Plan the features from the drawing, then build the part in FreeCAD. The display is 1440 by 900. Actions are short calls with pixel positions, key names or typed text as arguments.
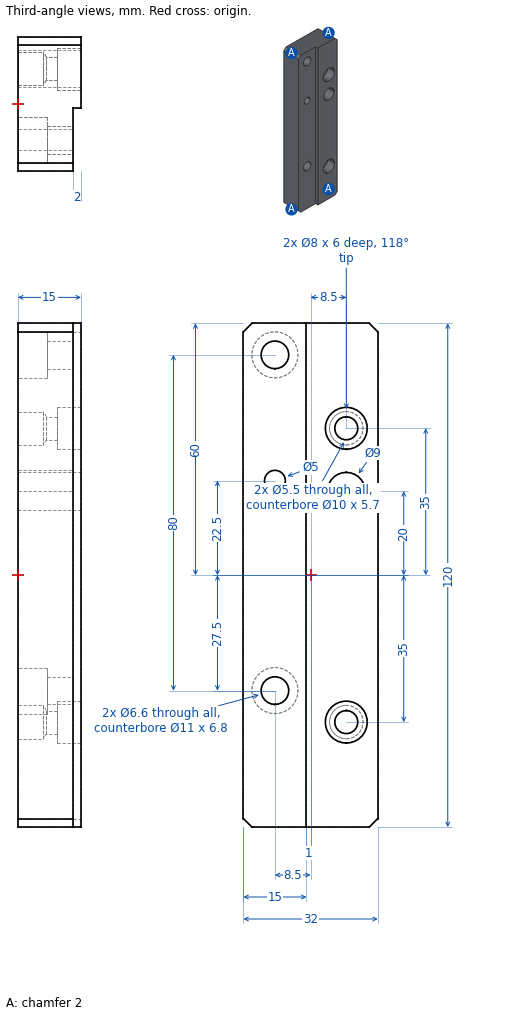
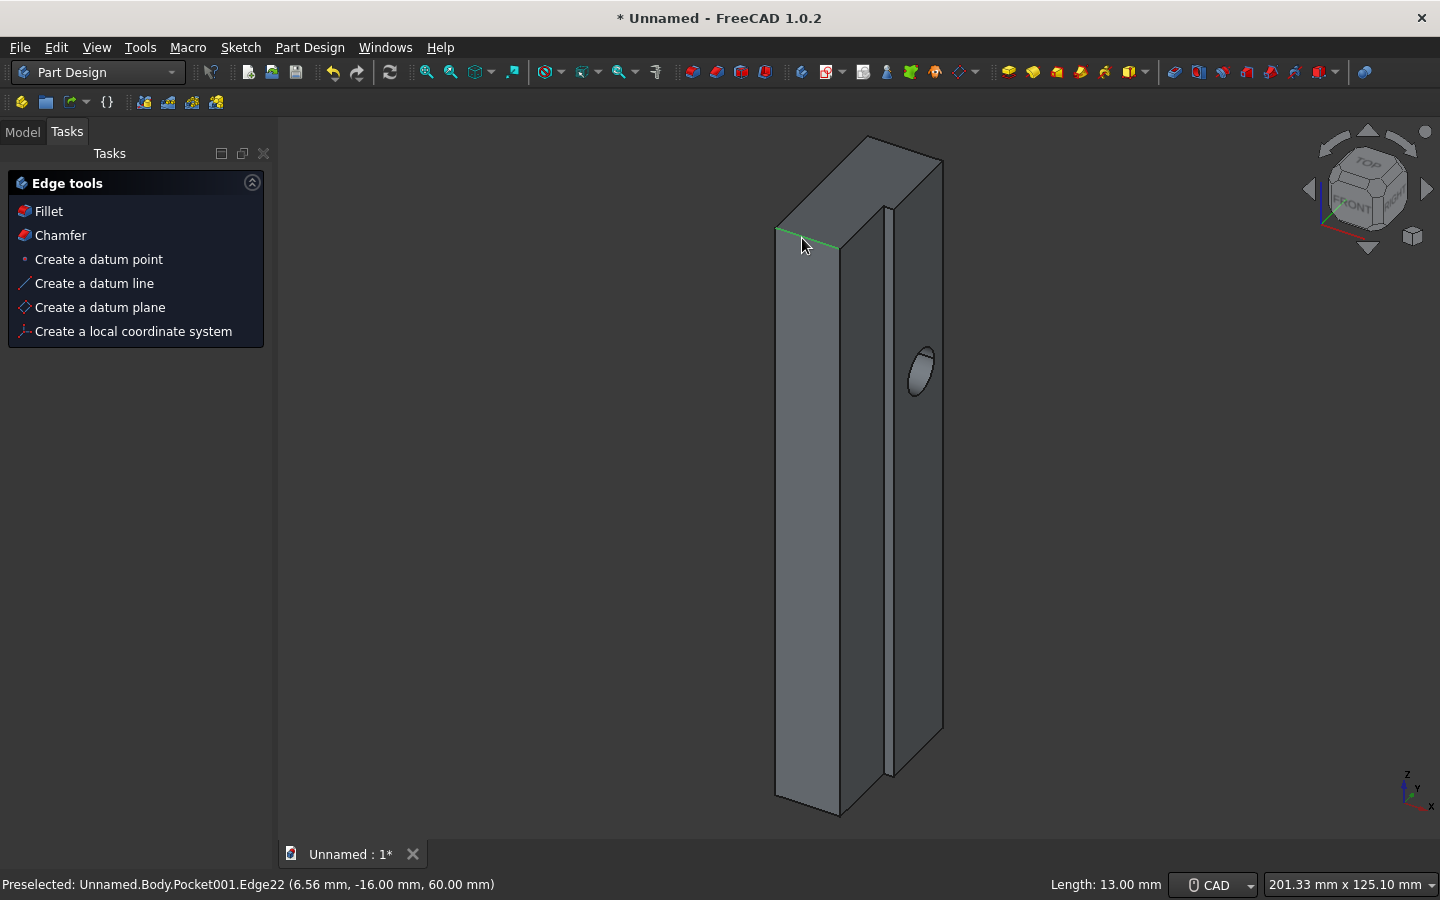
key(0)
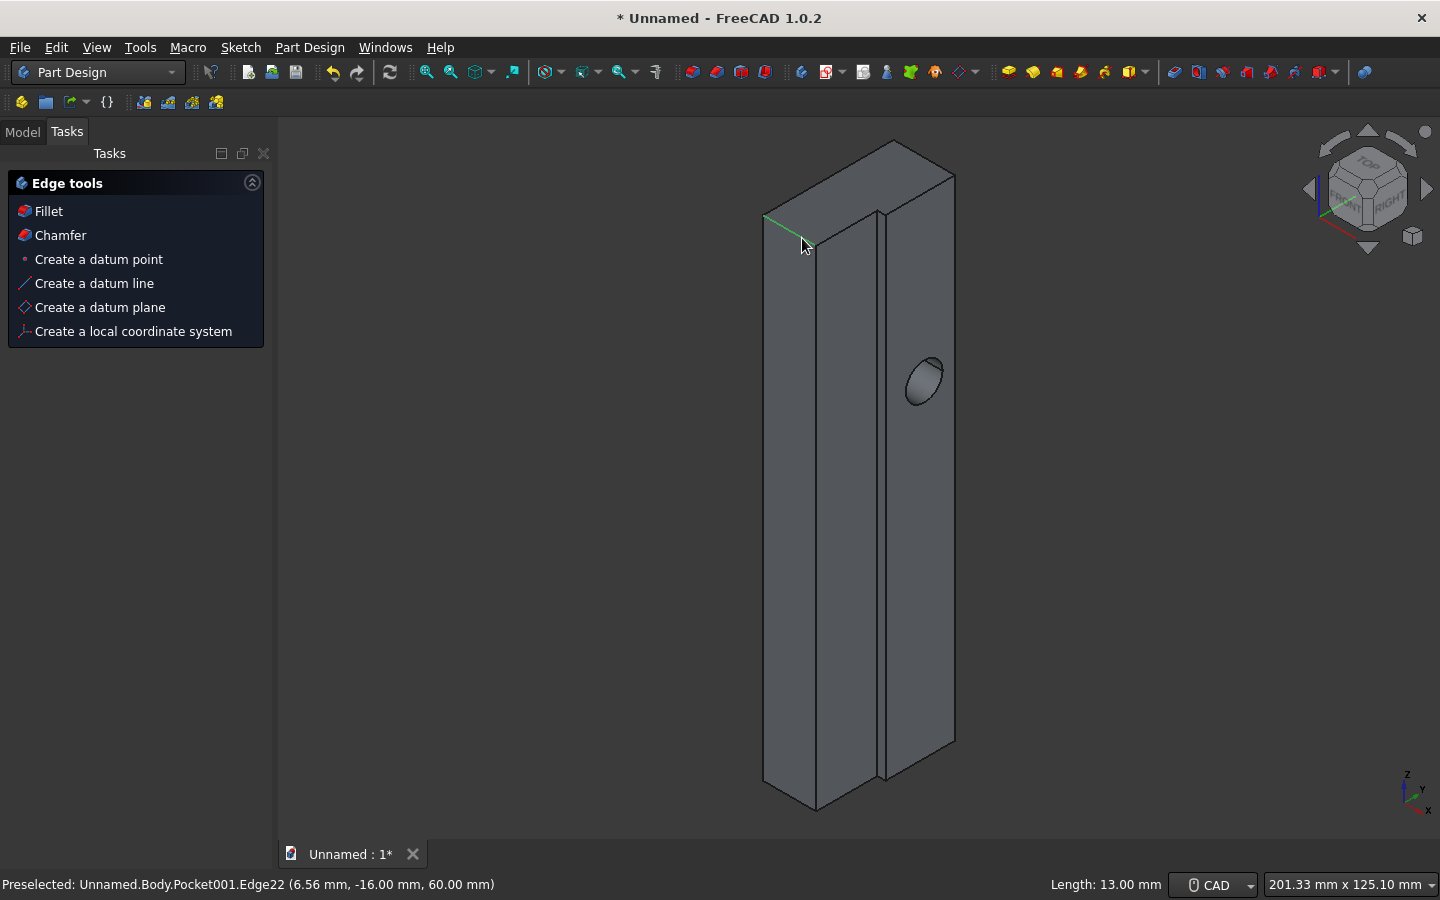
key(2)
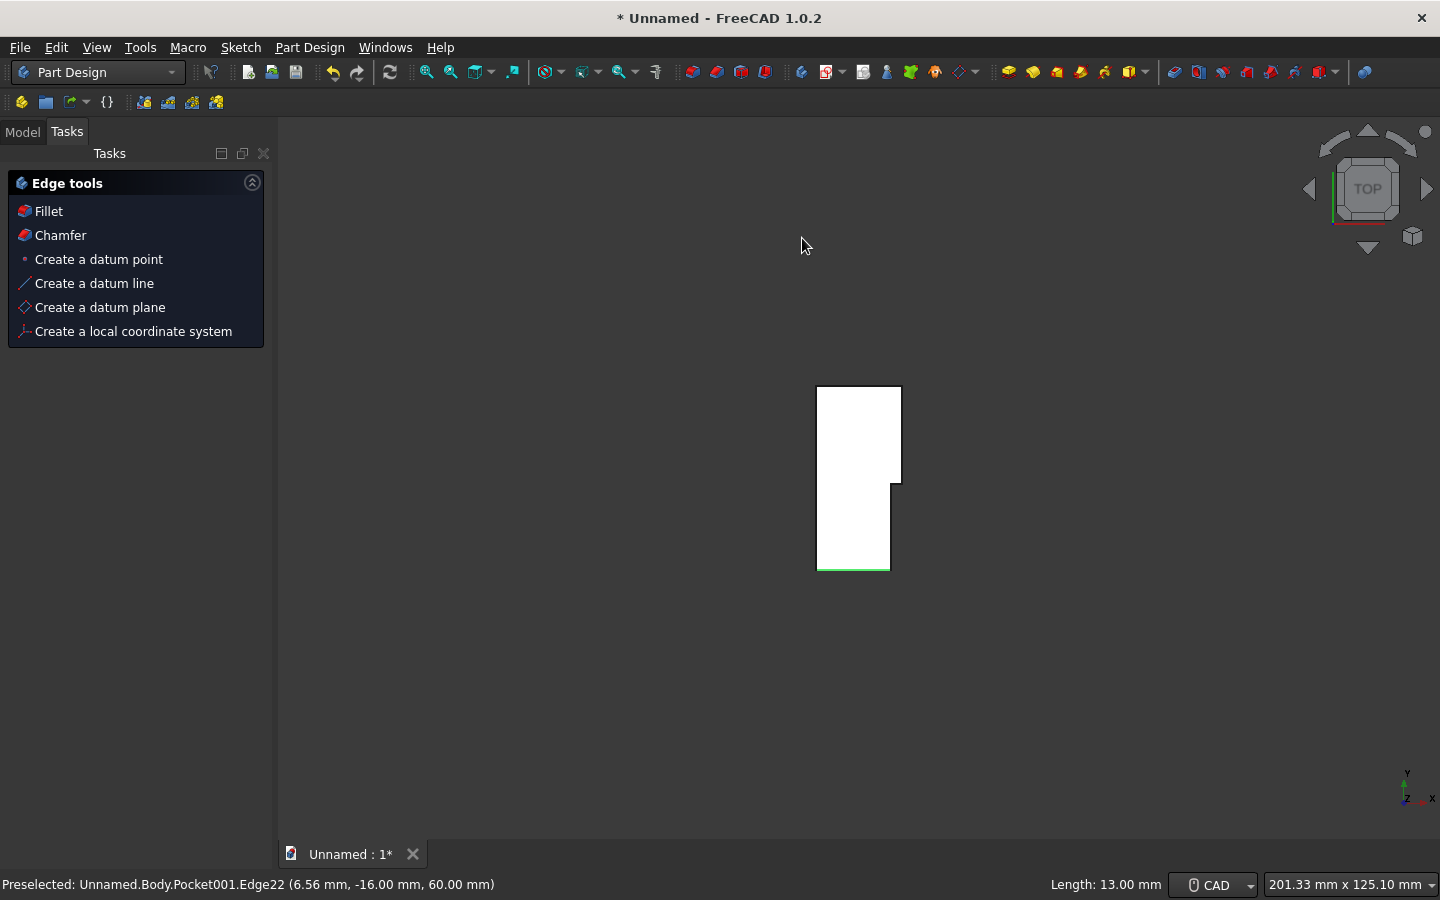
click(428, 72)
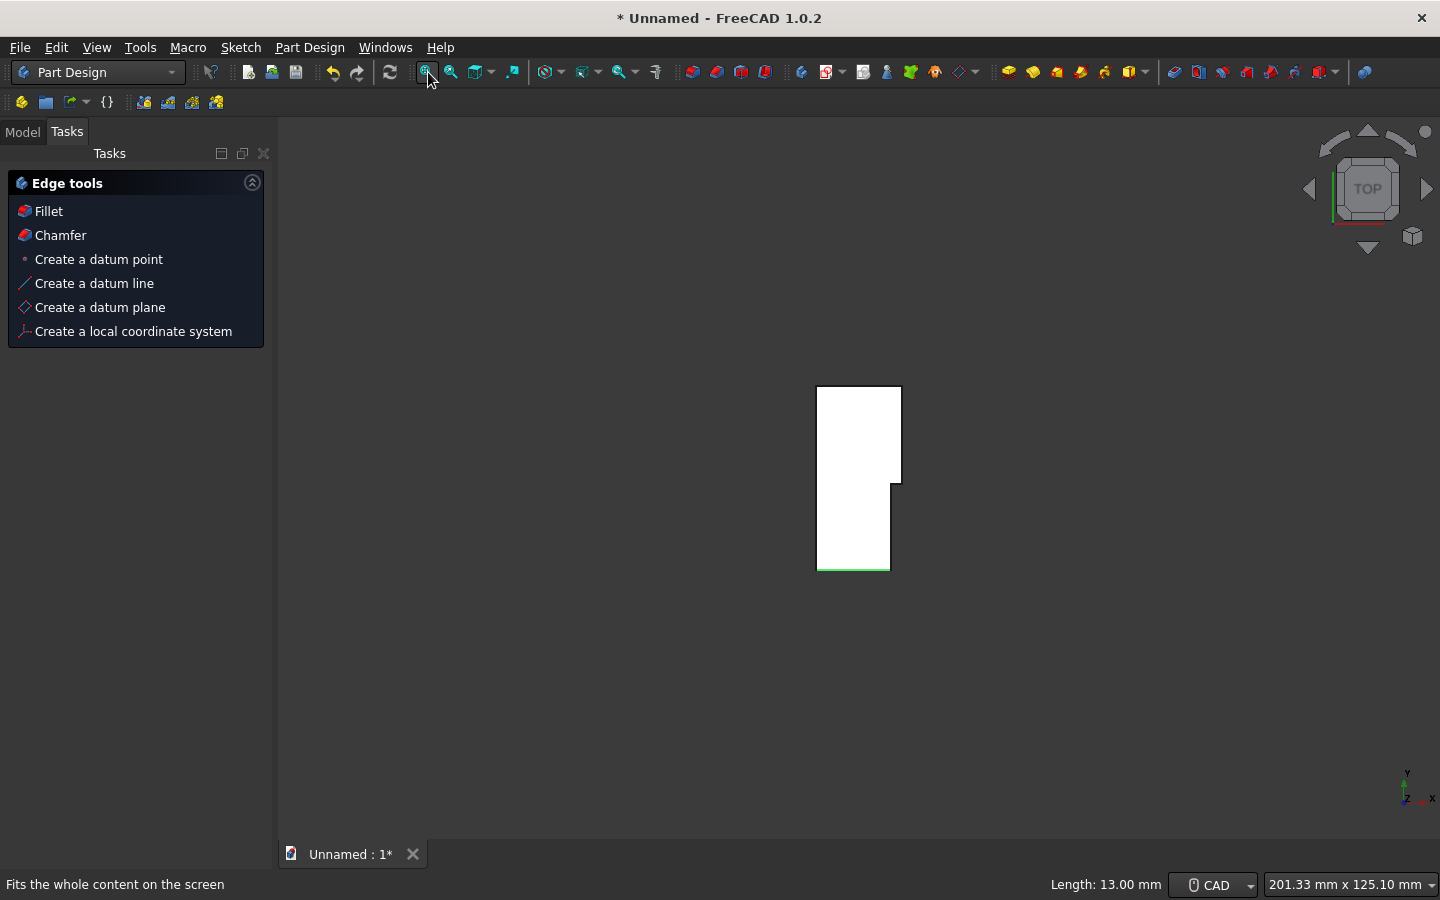
click(859, 385, ctrl)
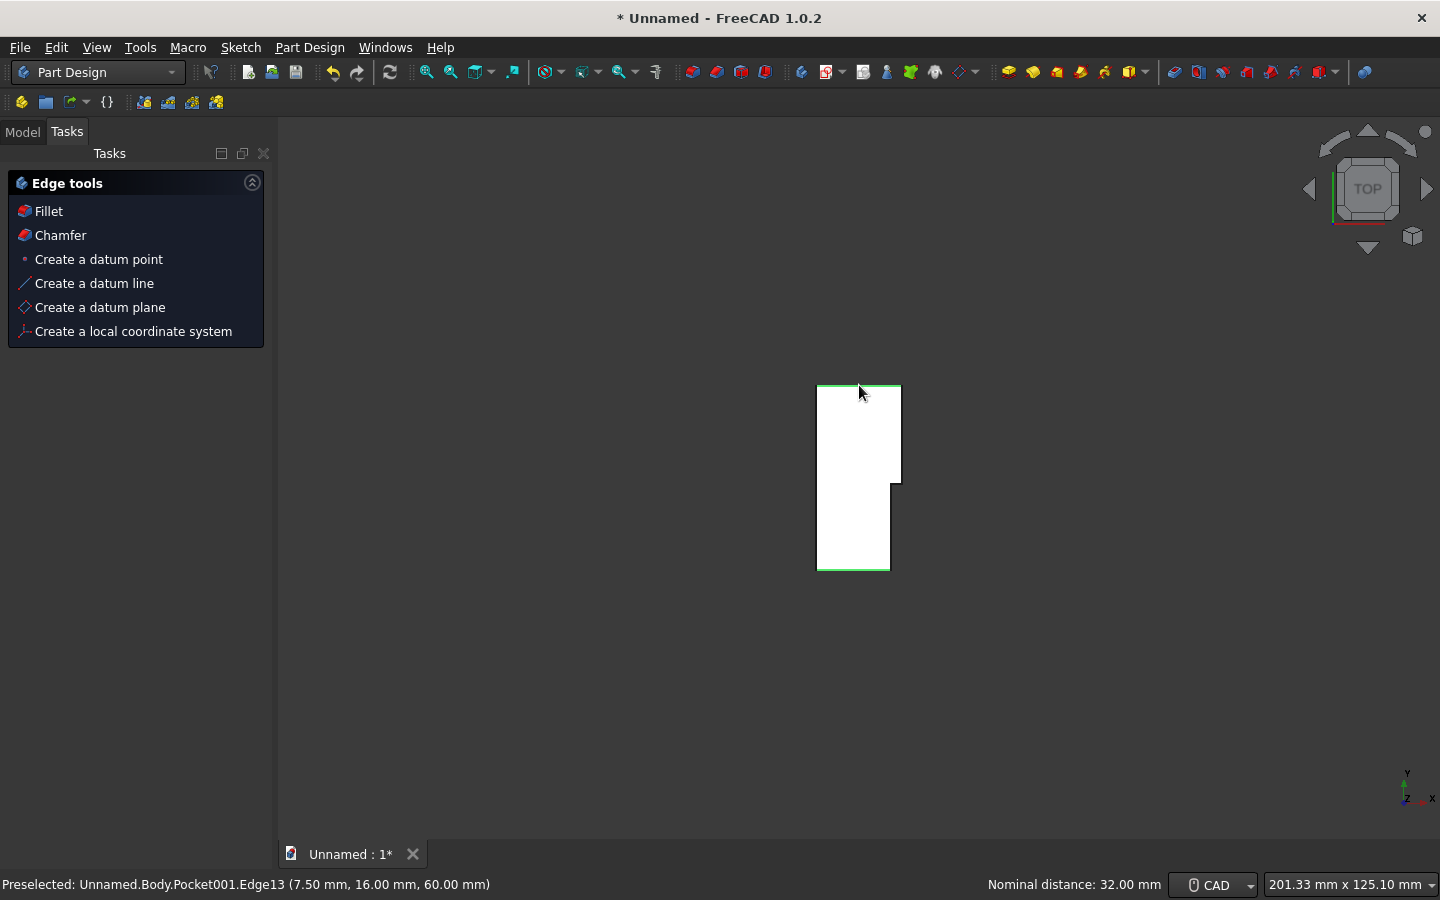
key(1)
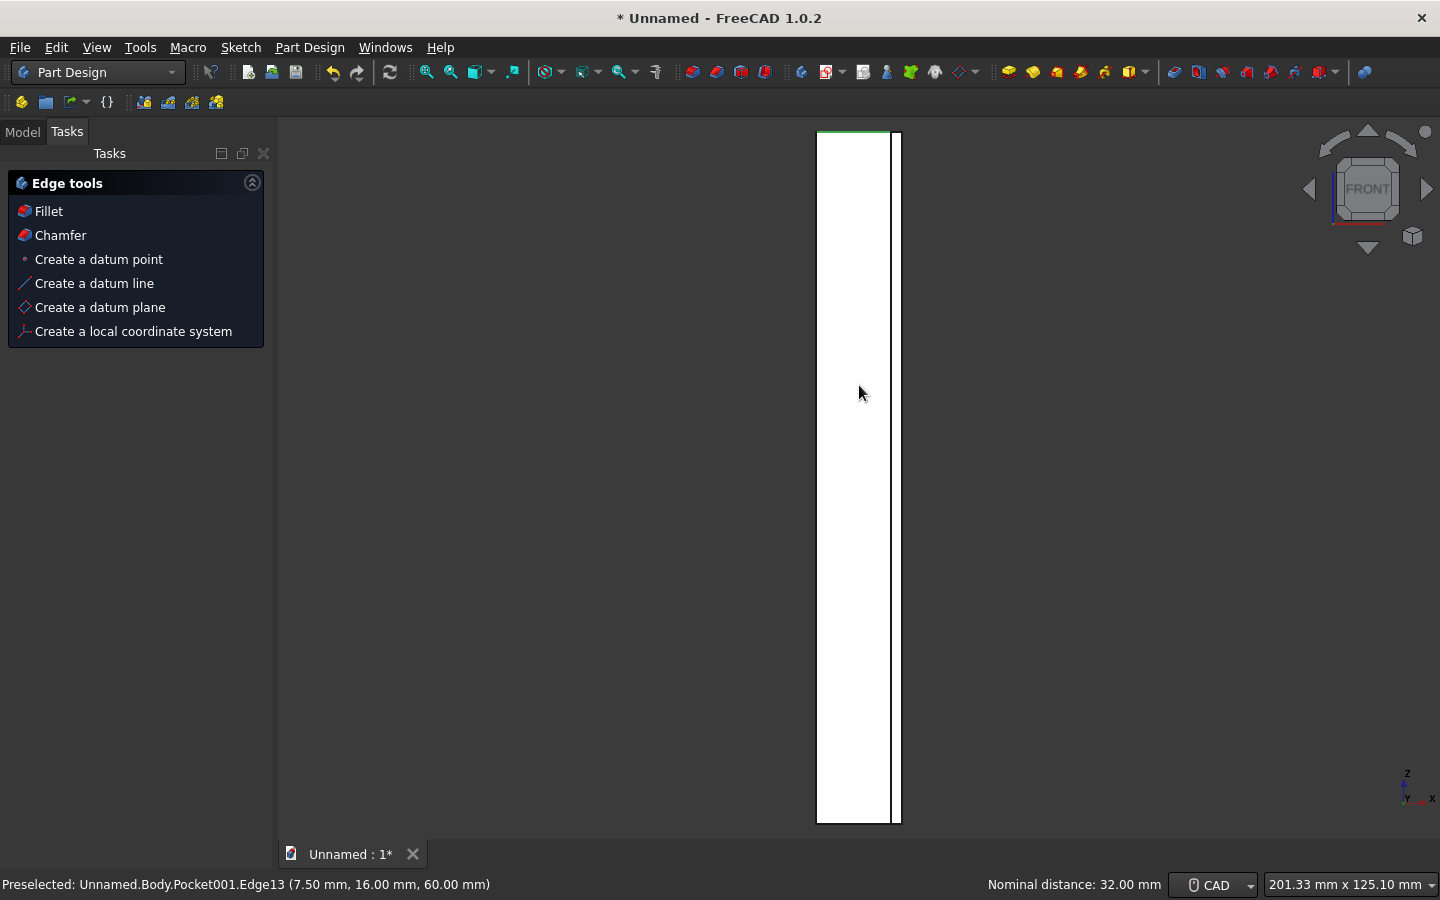
key(3)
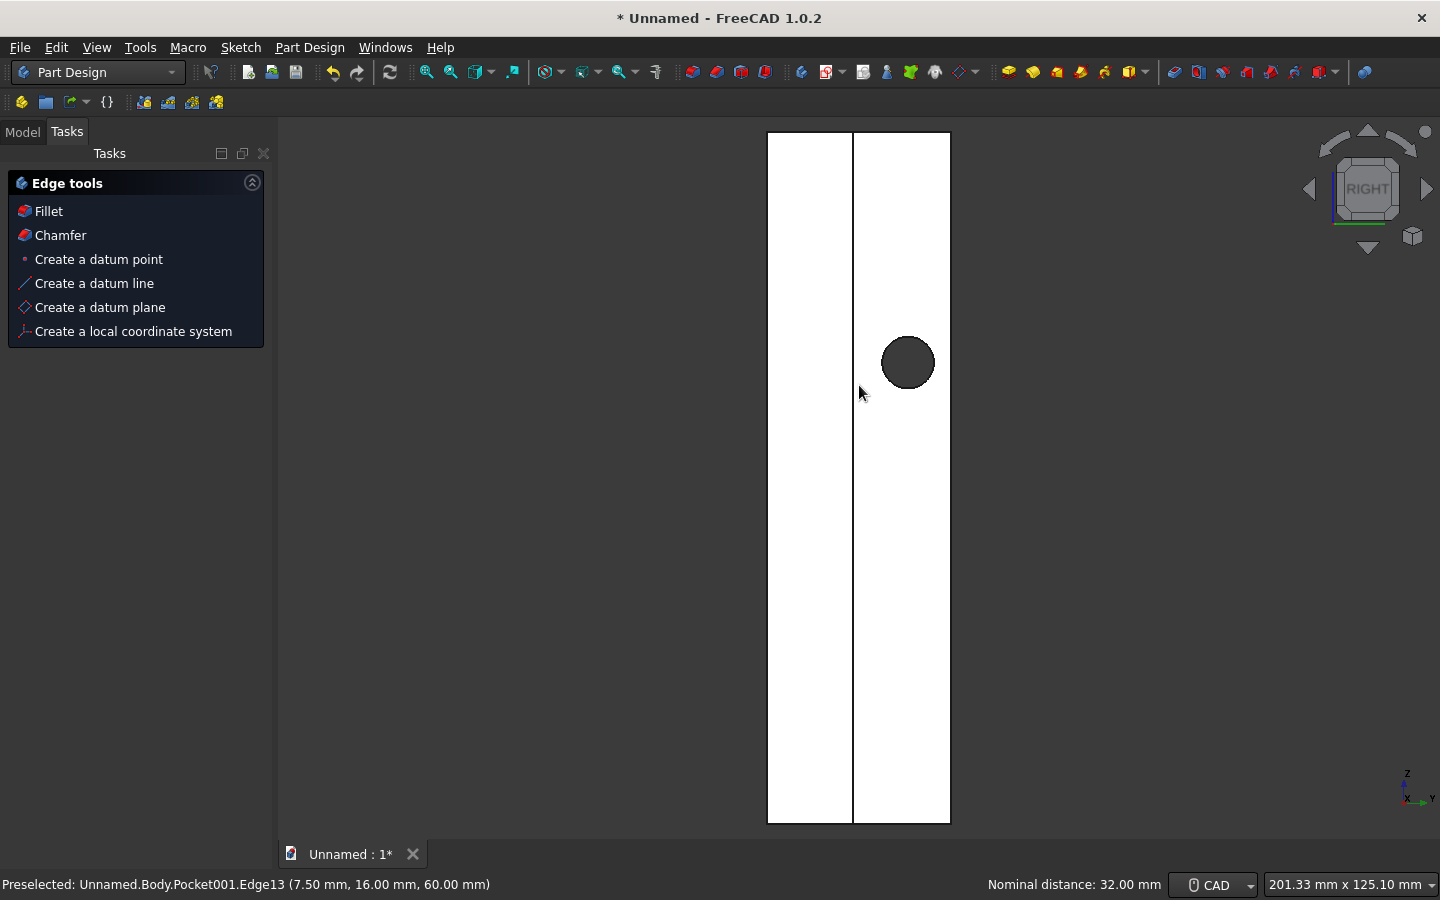
key(5)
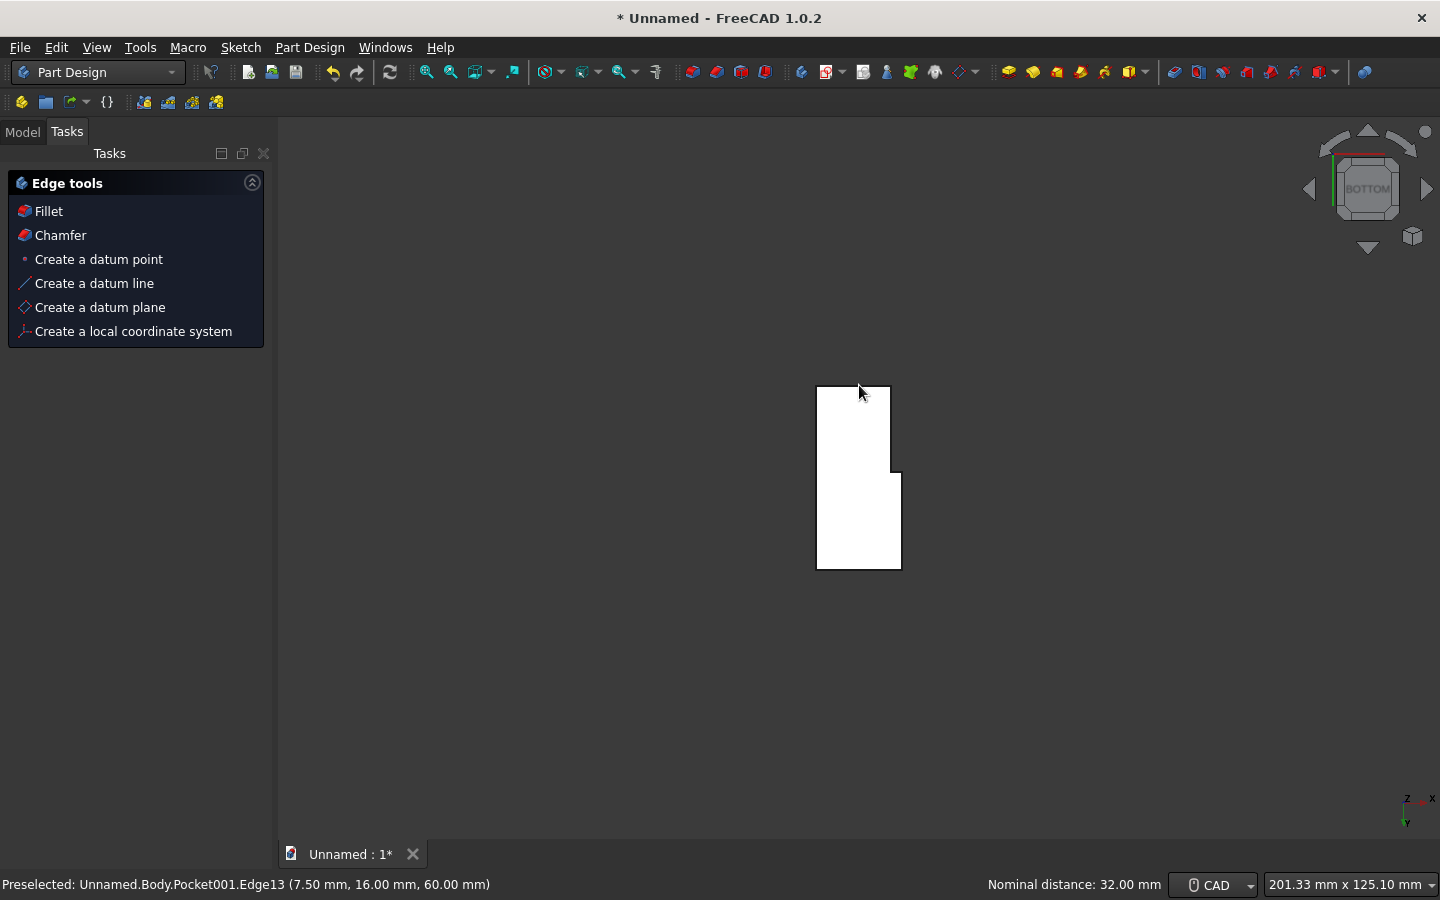
click(428, 72)